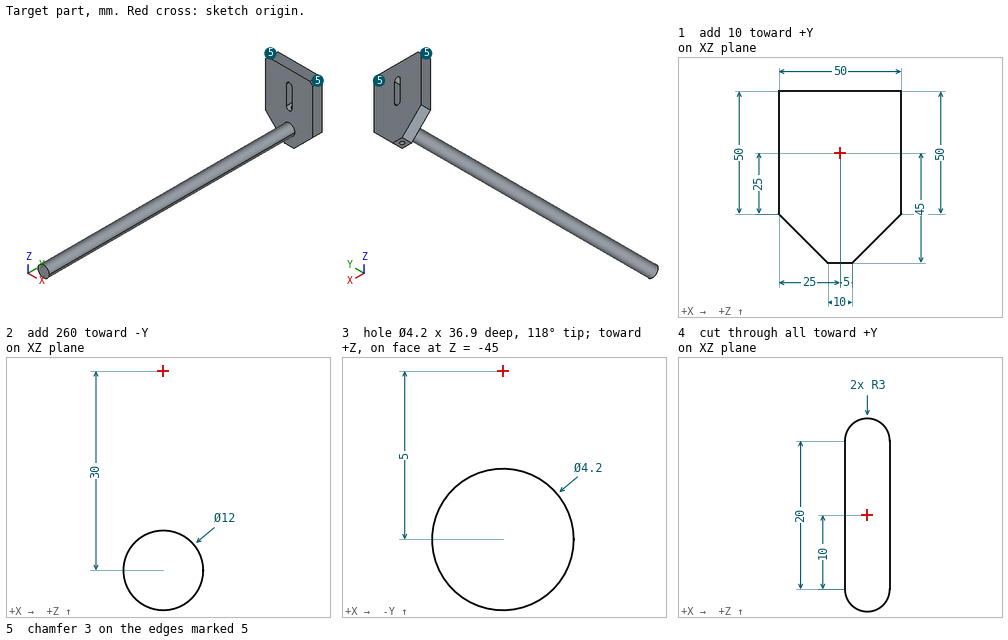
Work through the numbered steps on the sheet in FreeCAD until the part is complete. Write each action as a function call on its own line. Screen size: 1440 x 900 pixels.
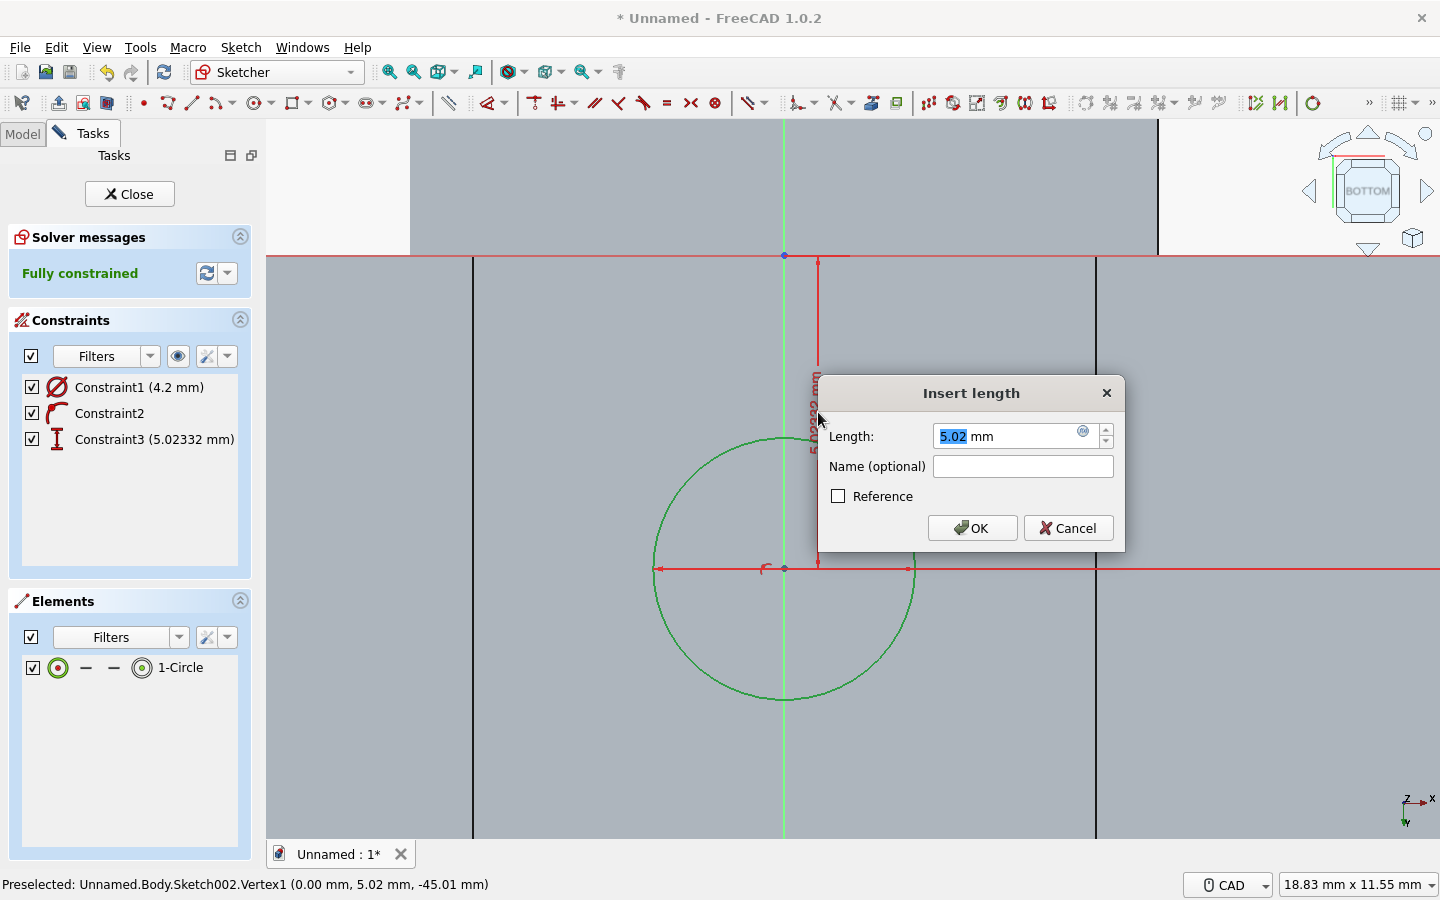
text(5)
key(Return)
key(Escape)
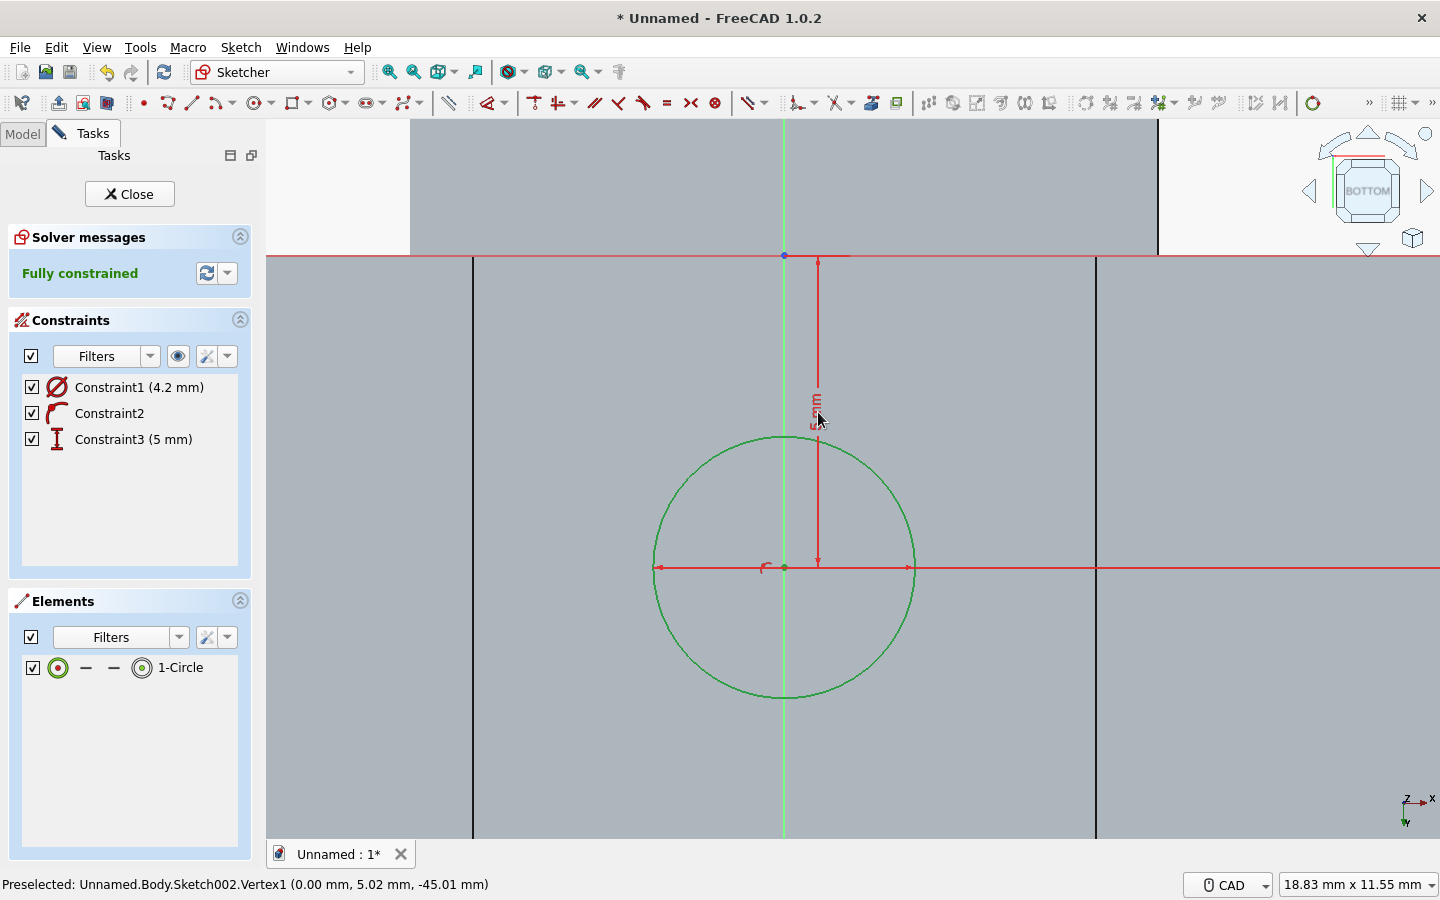
click(130, 194)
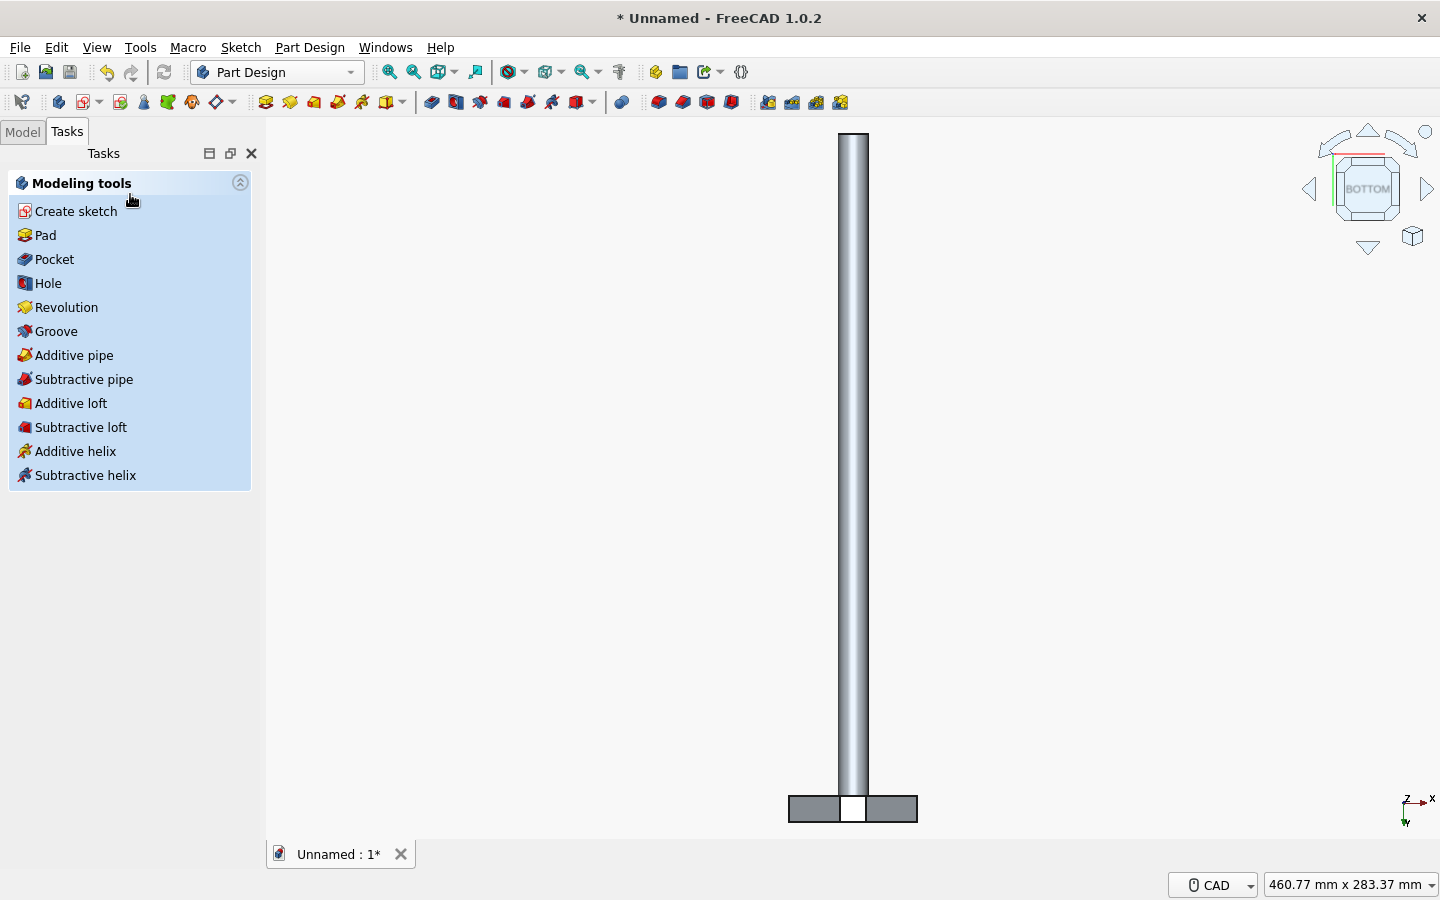
click(456, 102)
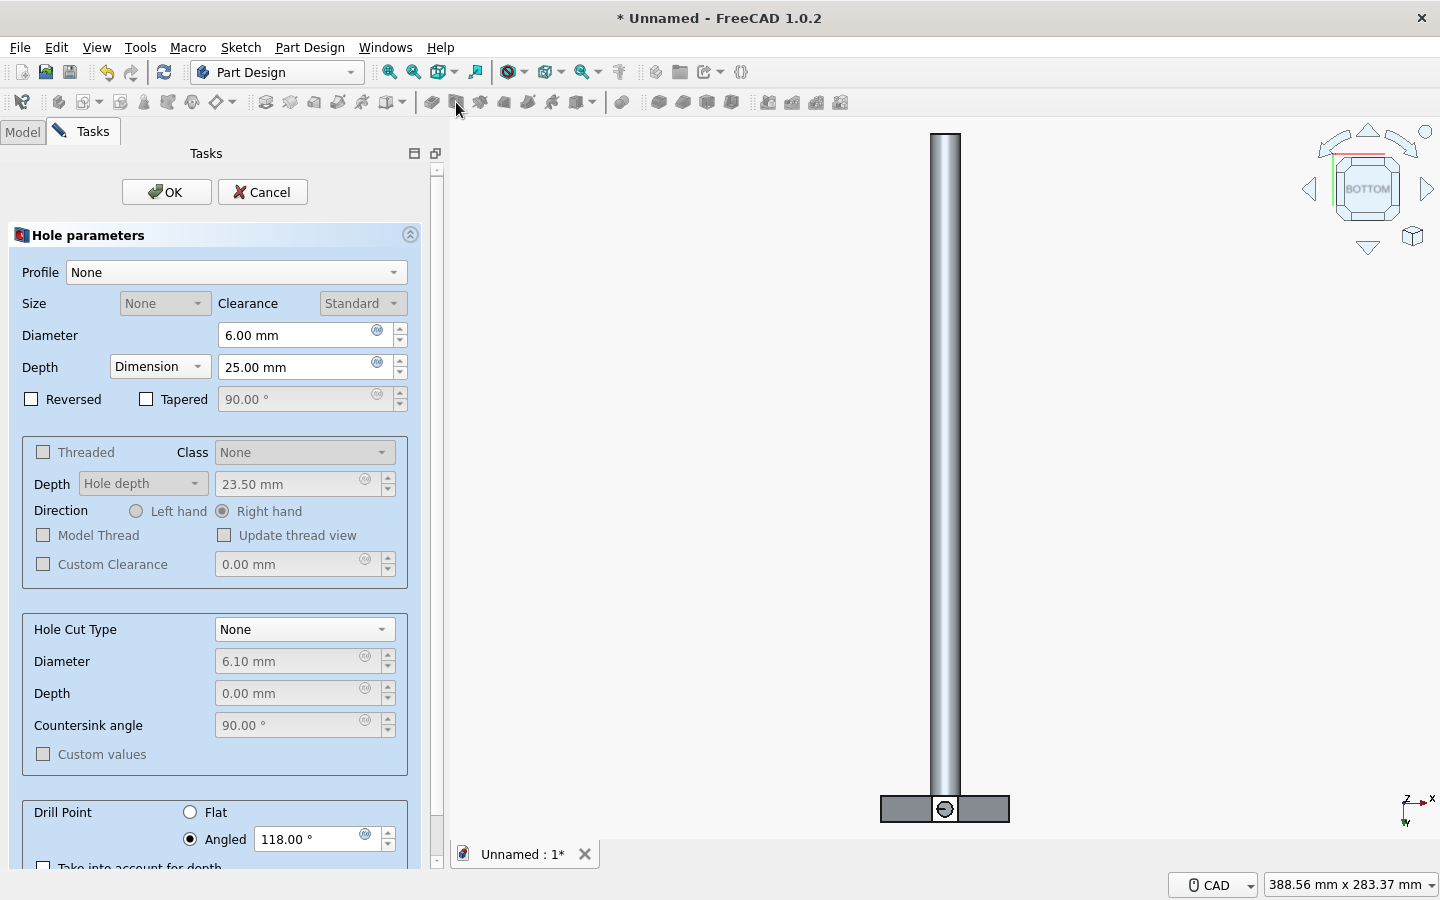
triple_click(305, 335)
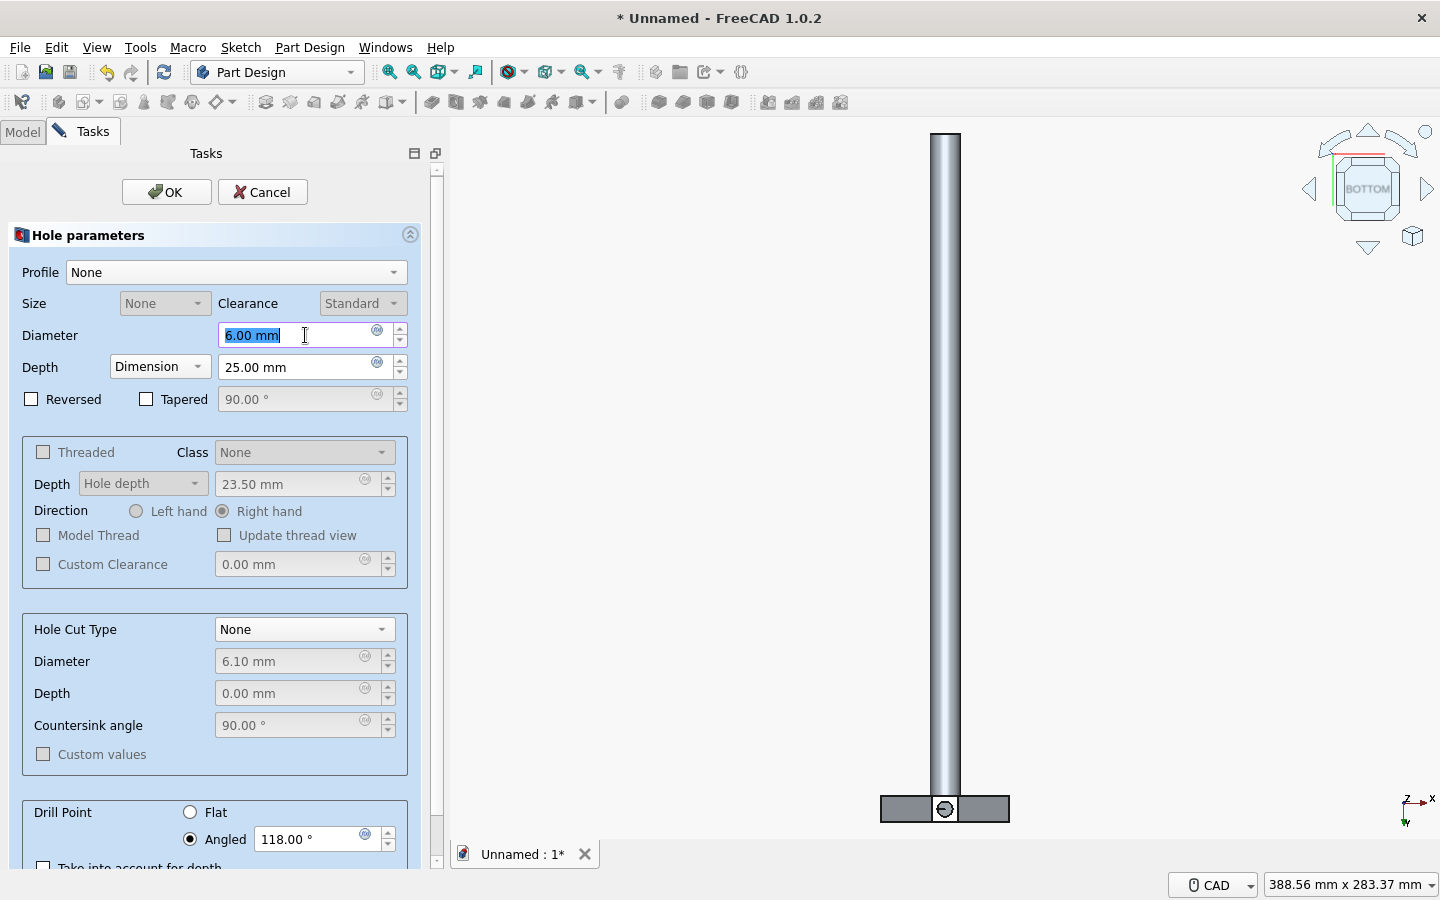
text(4.2)
key(Tab)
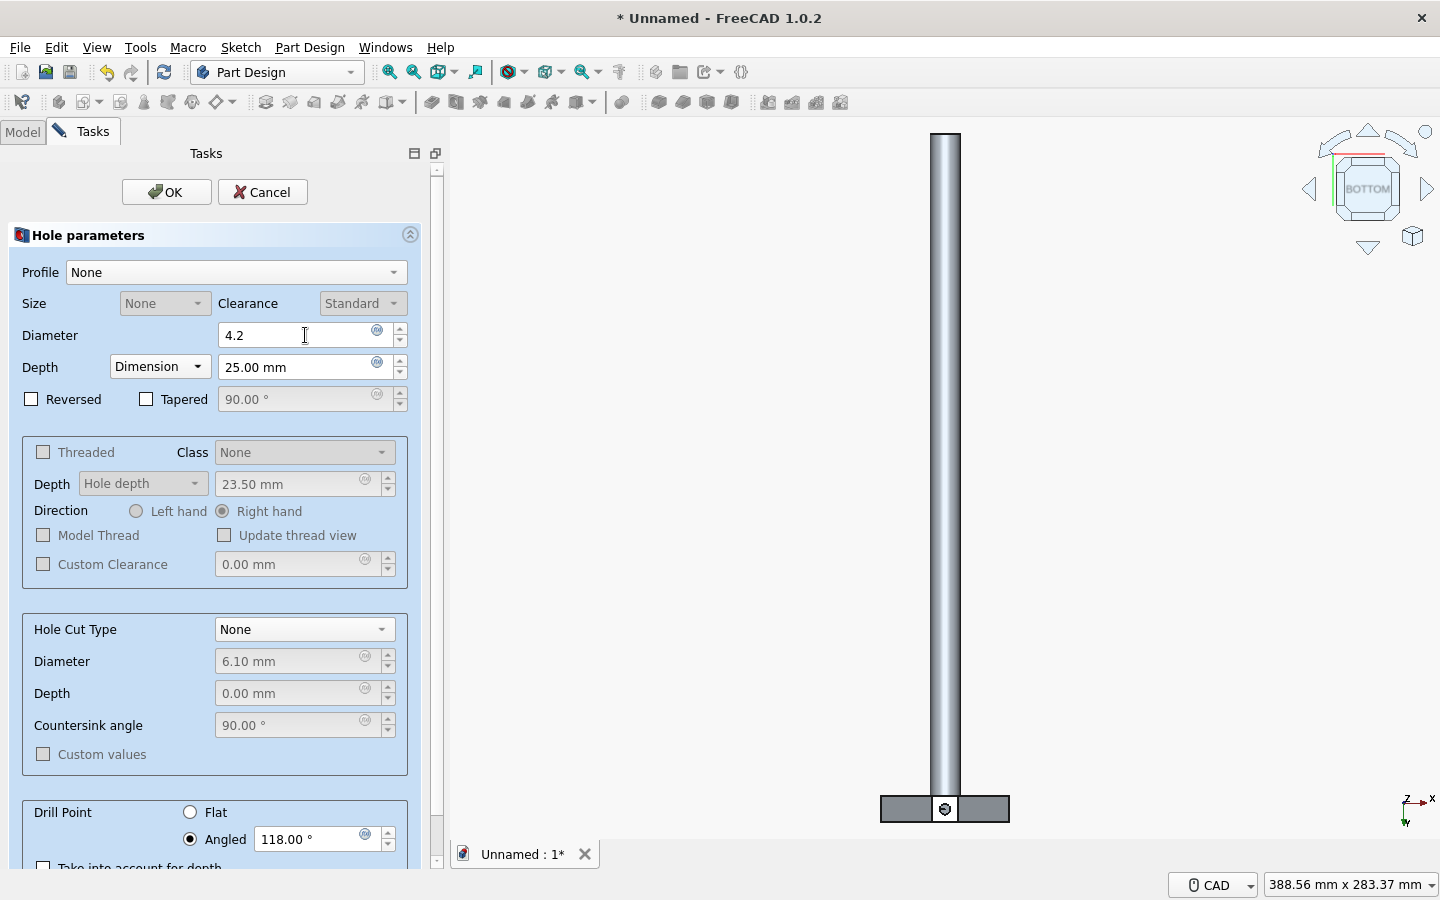
triple_click(305, 367)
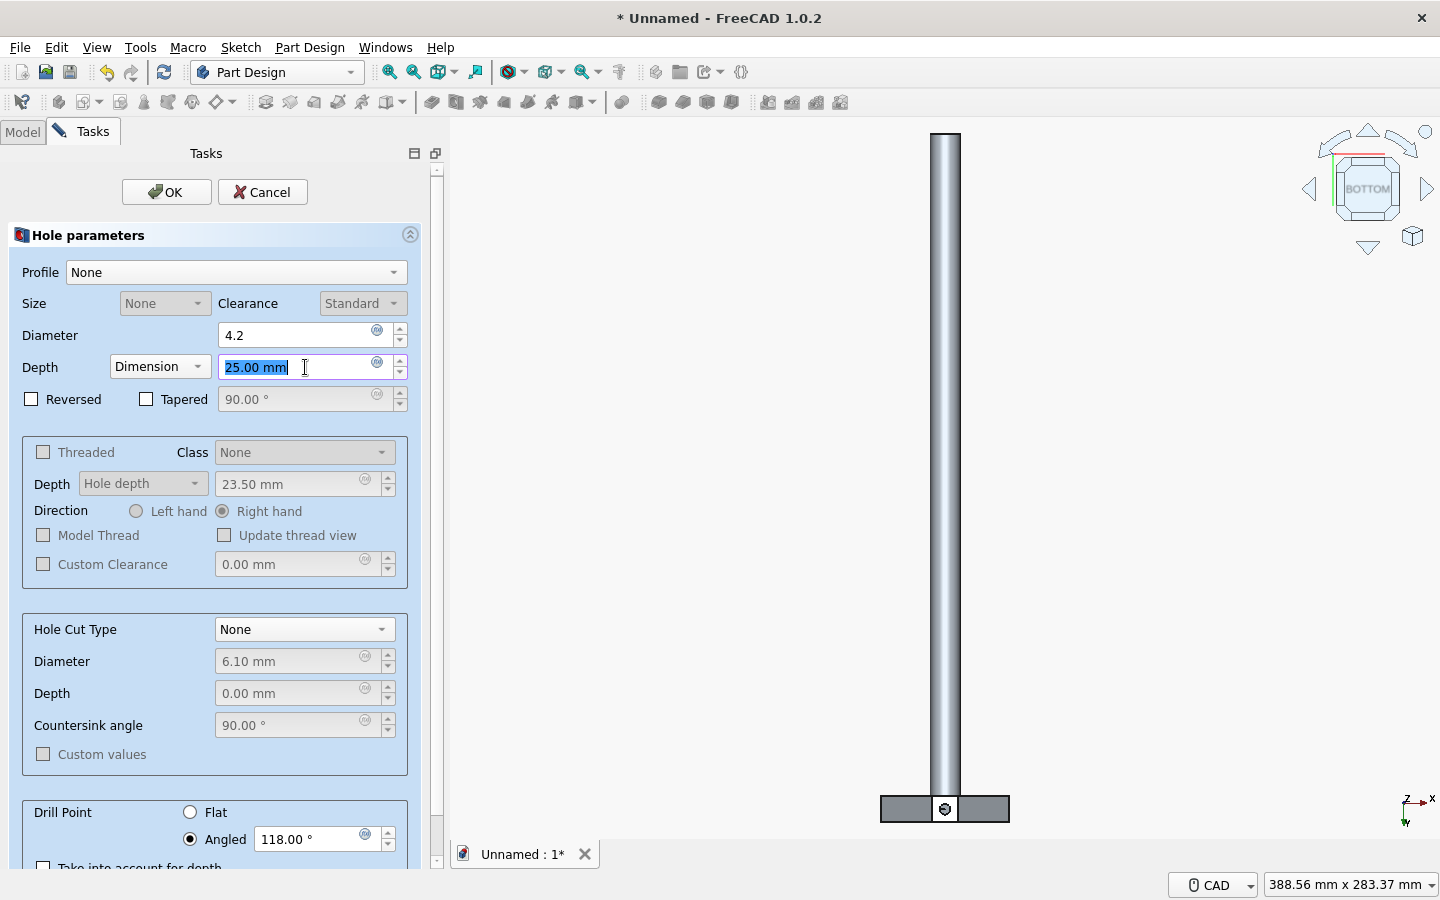
text(36.9)
key(Tab)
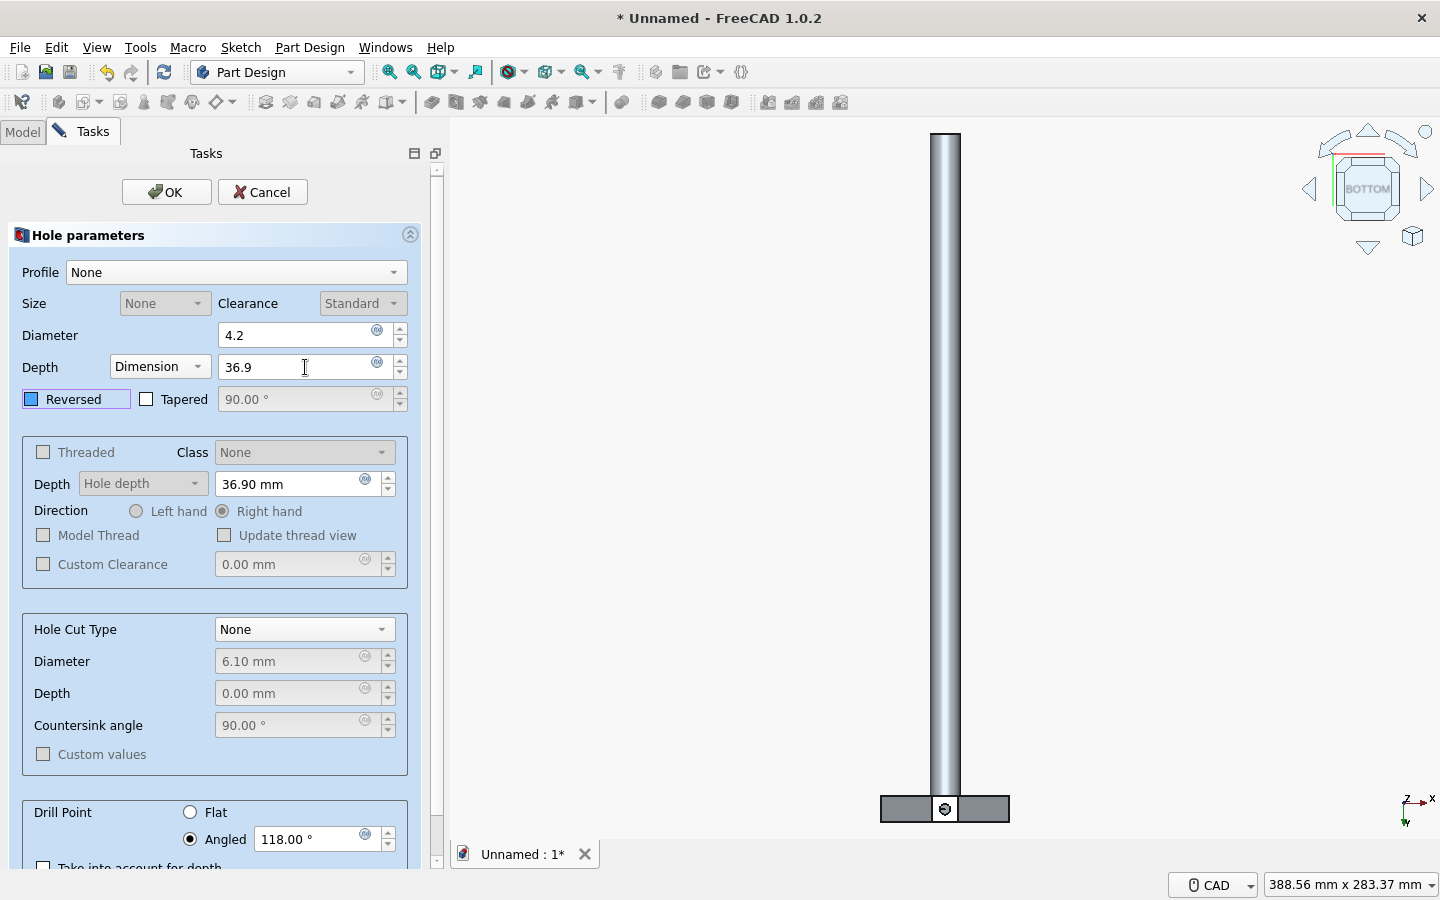
click(167, 192)